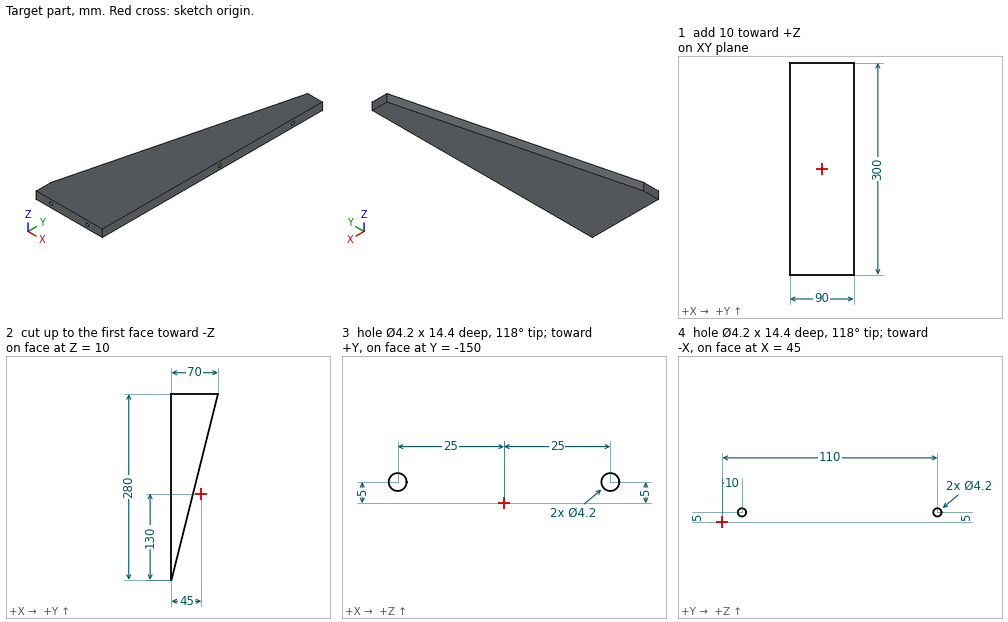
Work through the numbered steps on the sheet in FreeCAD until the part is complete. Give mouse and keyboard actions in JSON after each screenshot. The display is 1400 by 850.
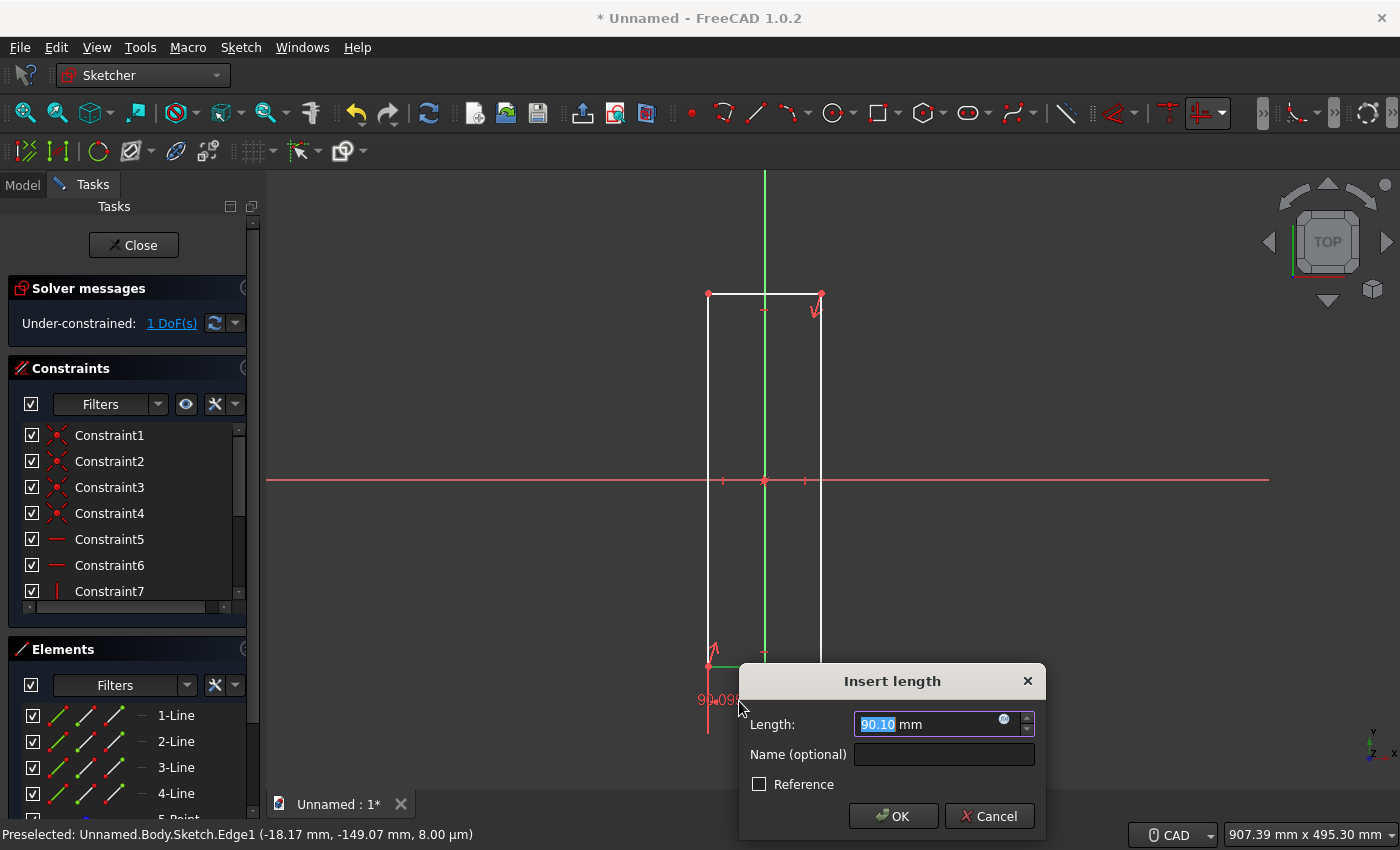
{"action": "type", "text": "90"}
{"action": "key", "text": "Return"}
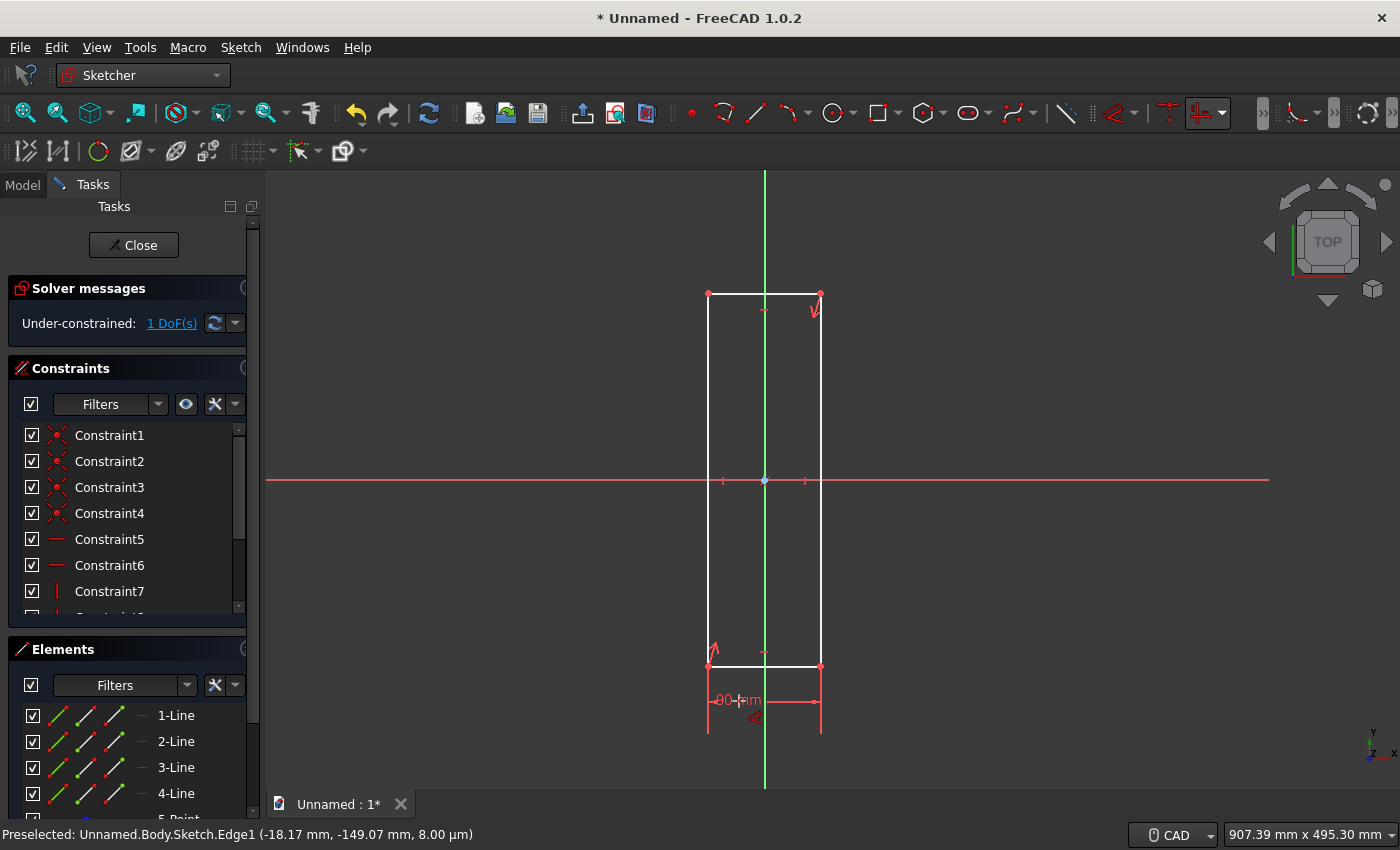
{"action": "left_click", "coordinate": [821, 555]}
{"action": "left_click", "coordinate": [855, 395]}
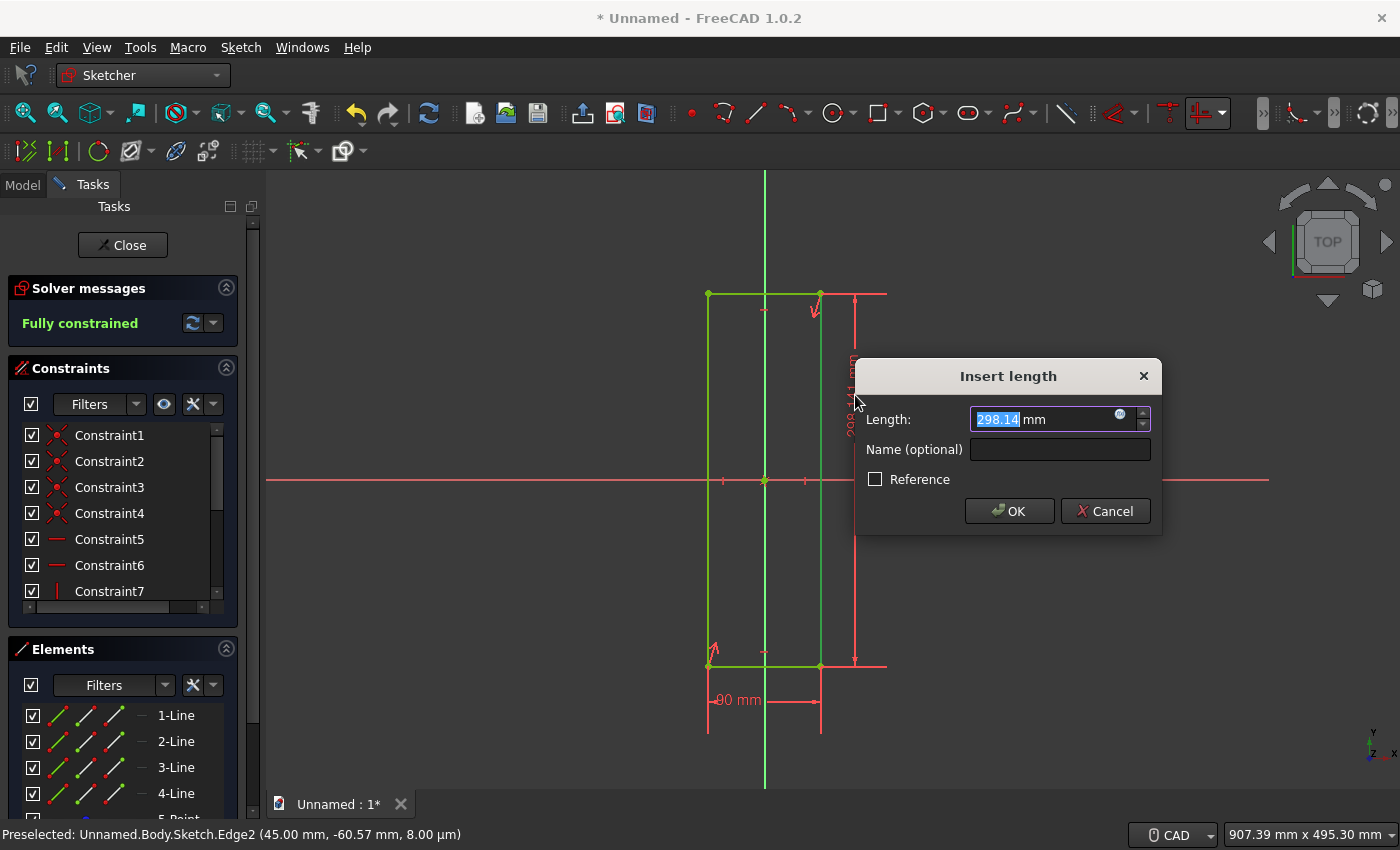
{"action": "type", "text": "300"}
{"action": "key", "text": "Return"}
{"action": "key", "text": "Escape"}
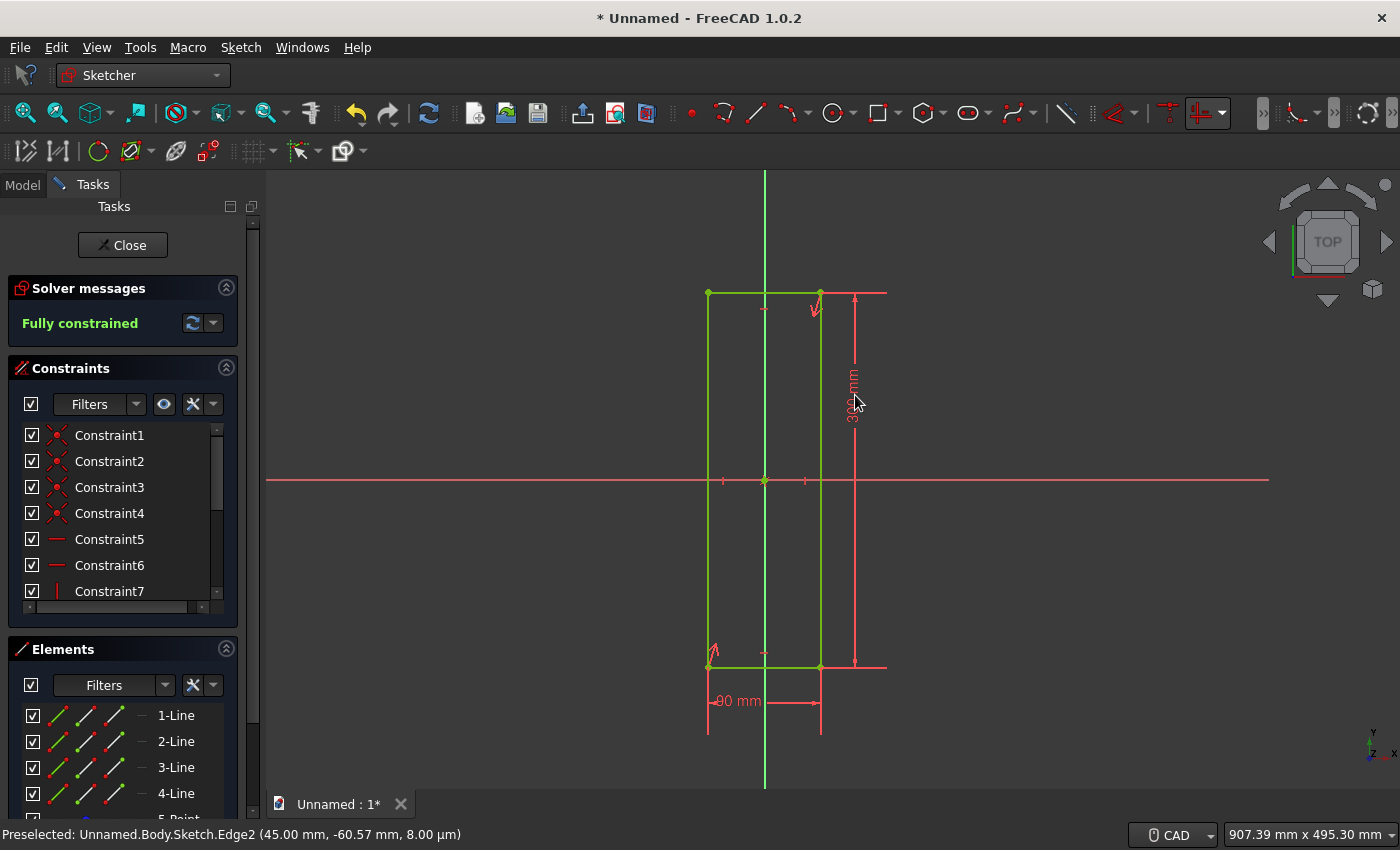
{"action": "left_click", "coordinate": [123, 245]}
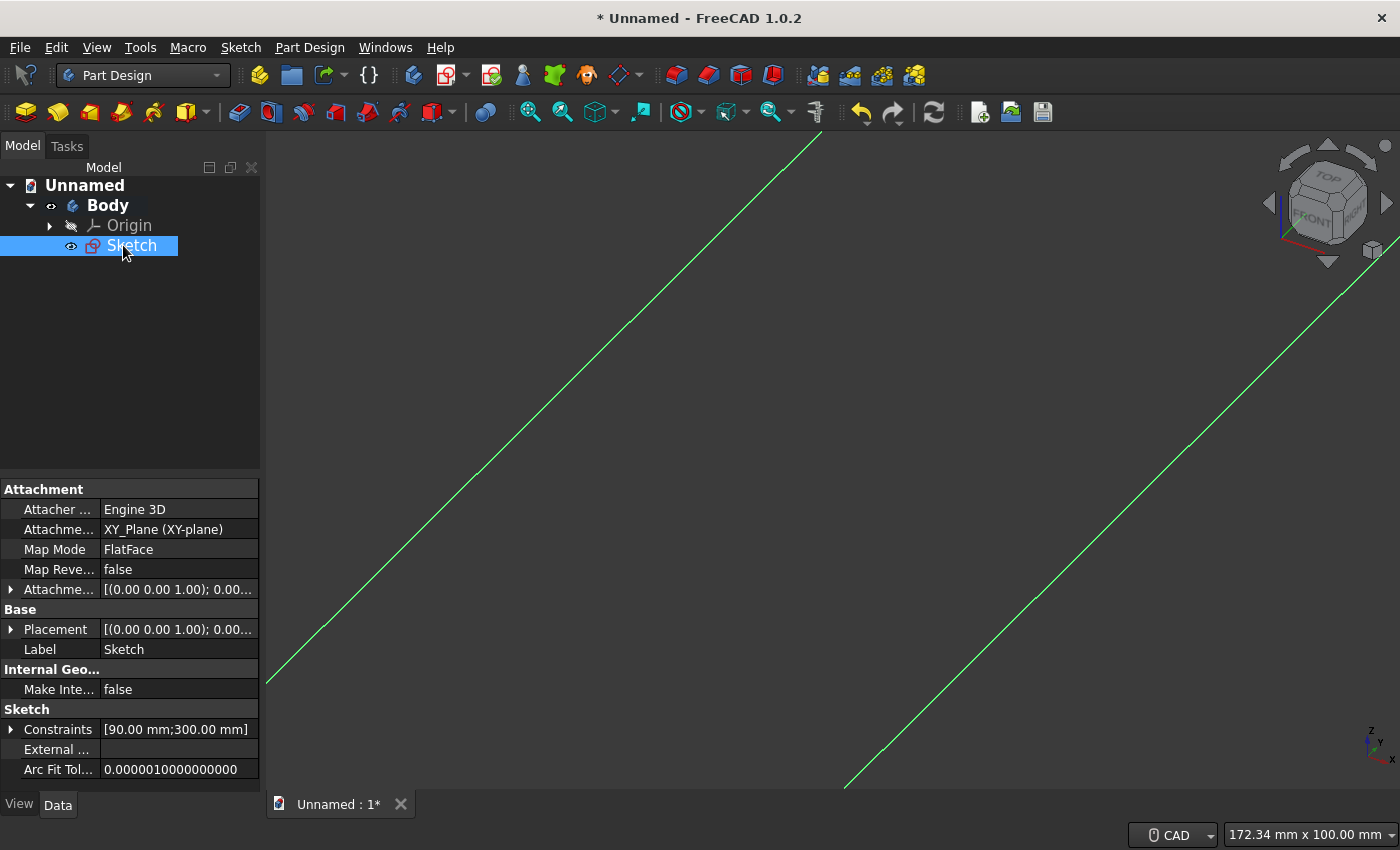
{"action": "left_click", "coordinate": [26, 112]}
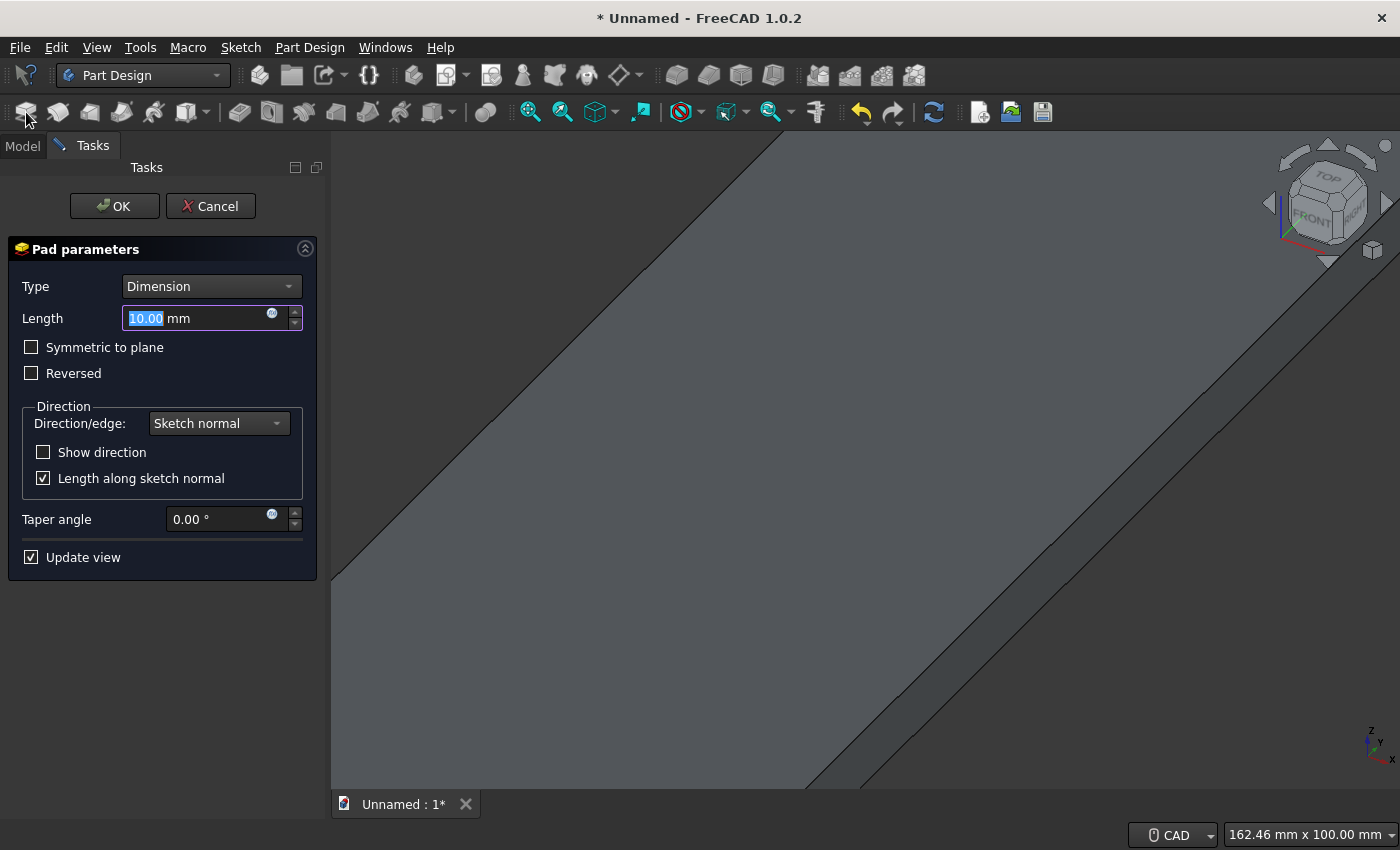
{"action": "type", "text": "10"}
{"action": "key", "text": "Tab"}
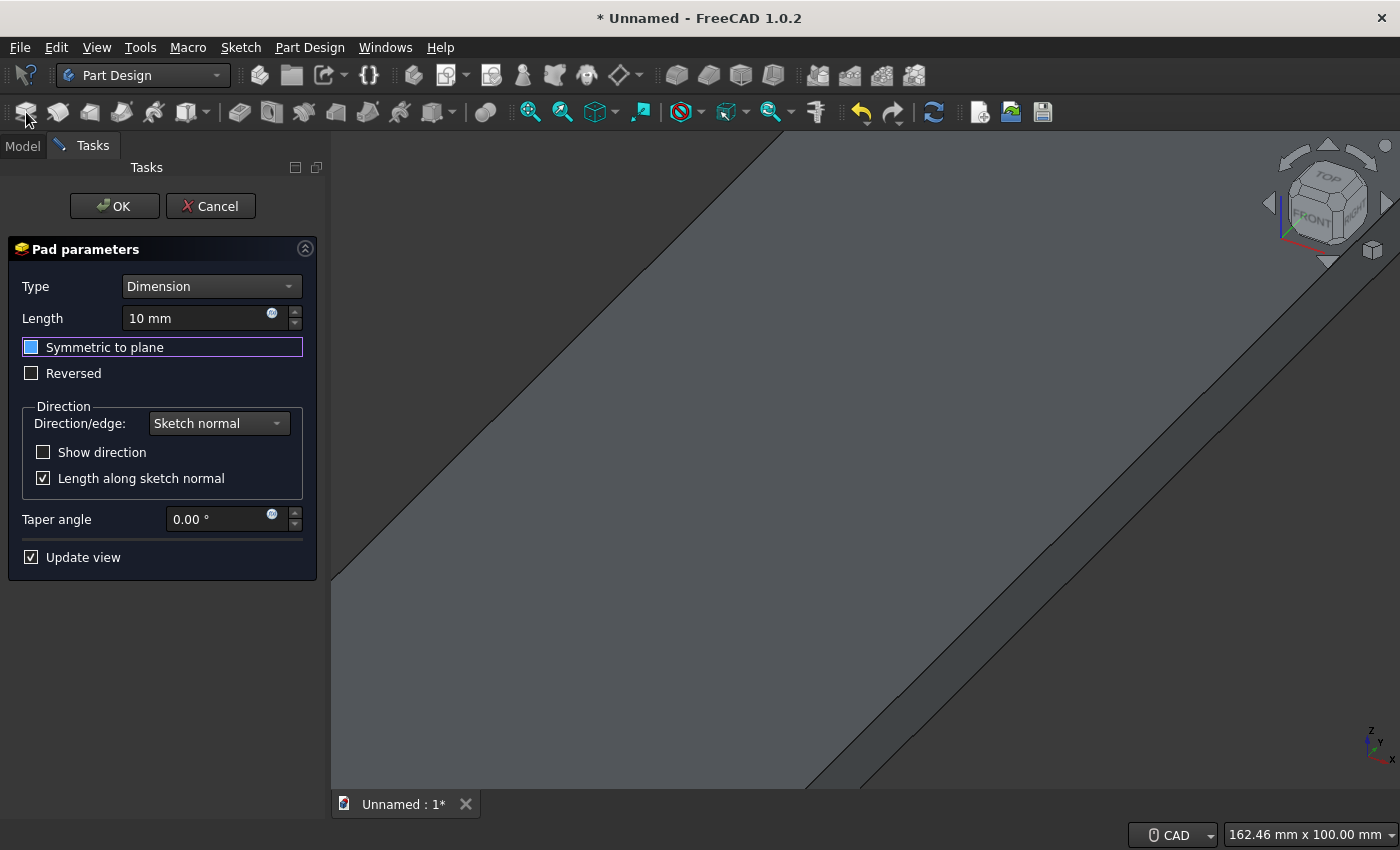
{"action": "left_click", "coordinate": [115, 206]}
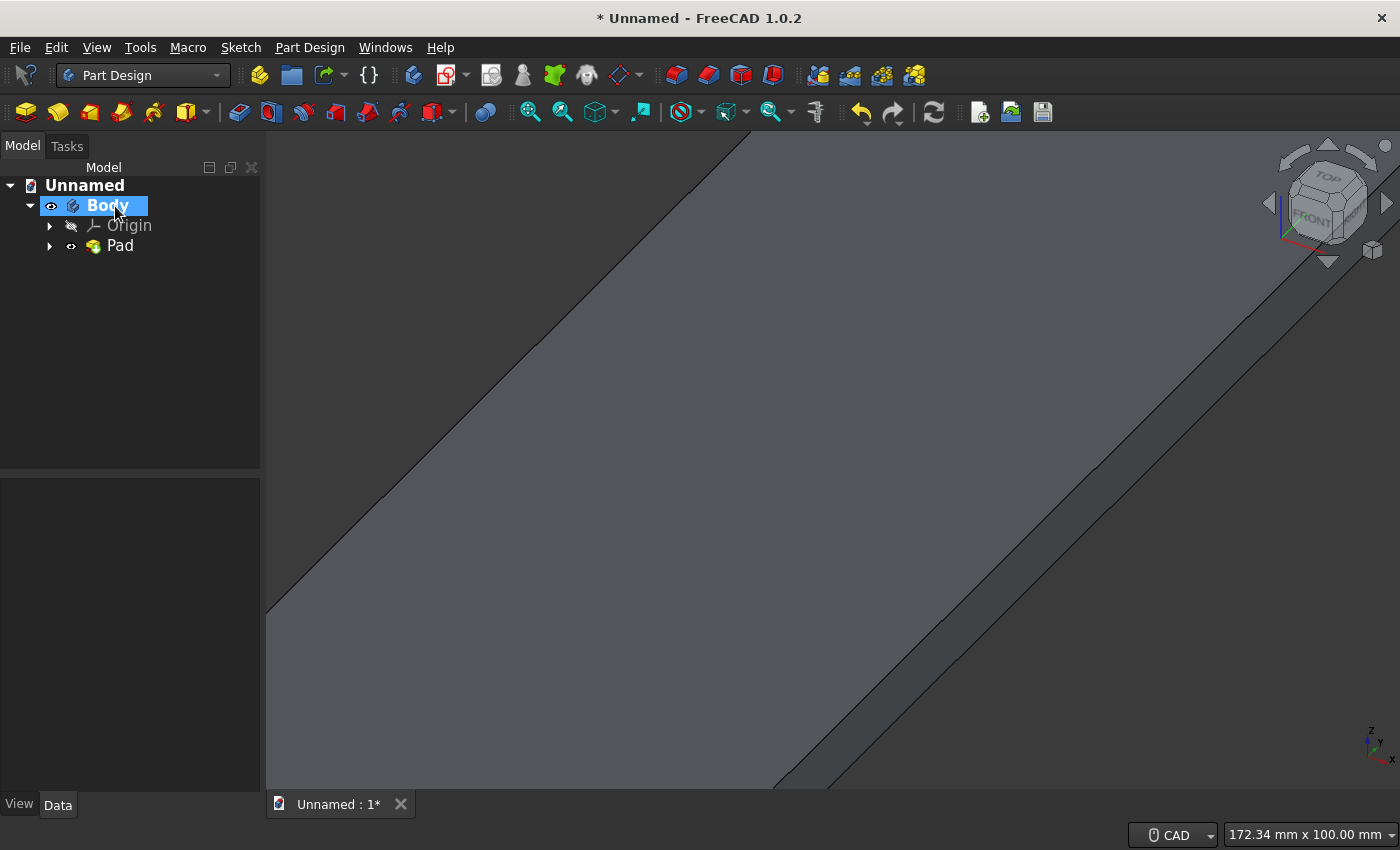
{"action": "key", "text": "v f"}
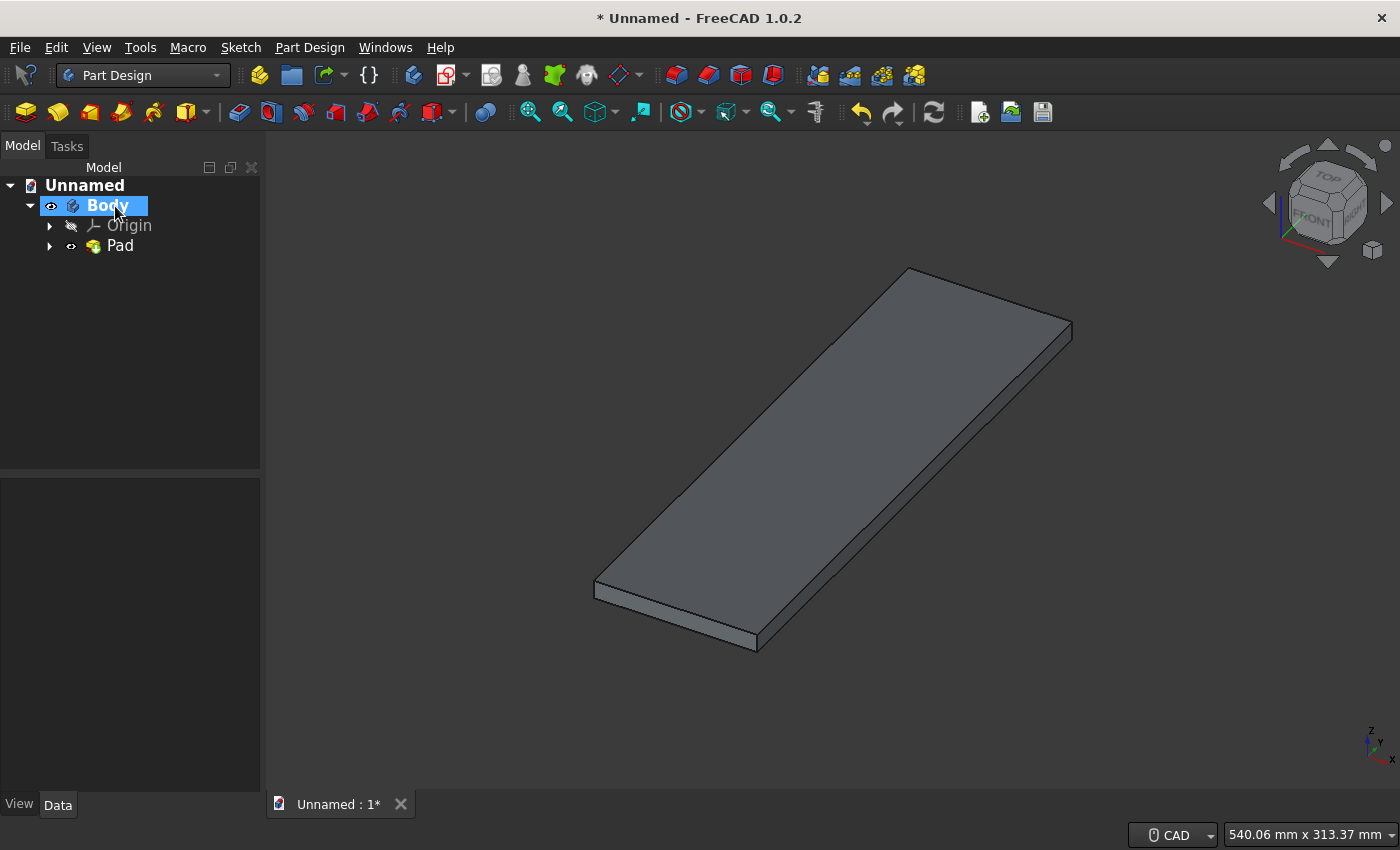
{"action": "left_click", "coordinate": [923, 361]}